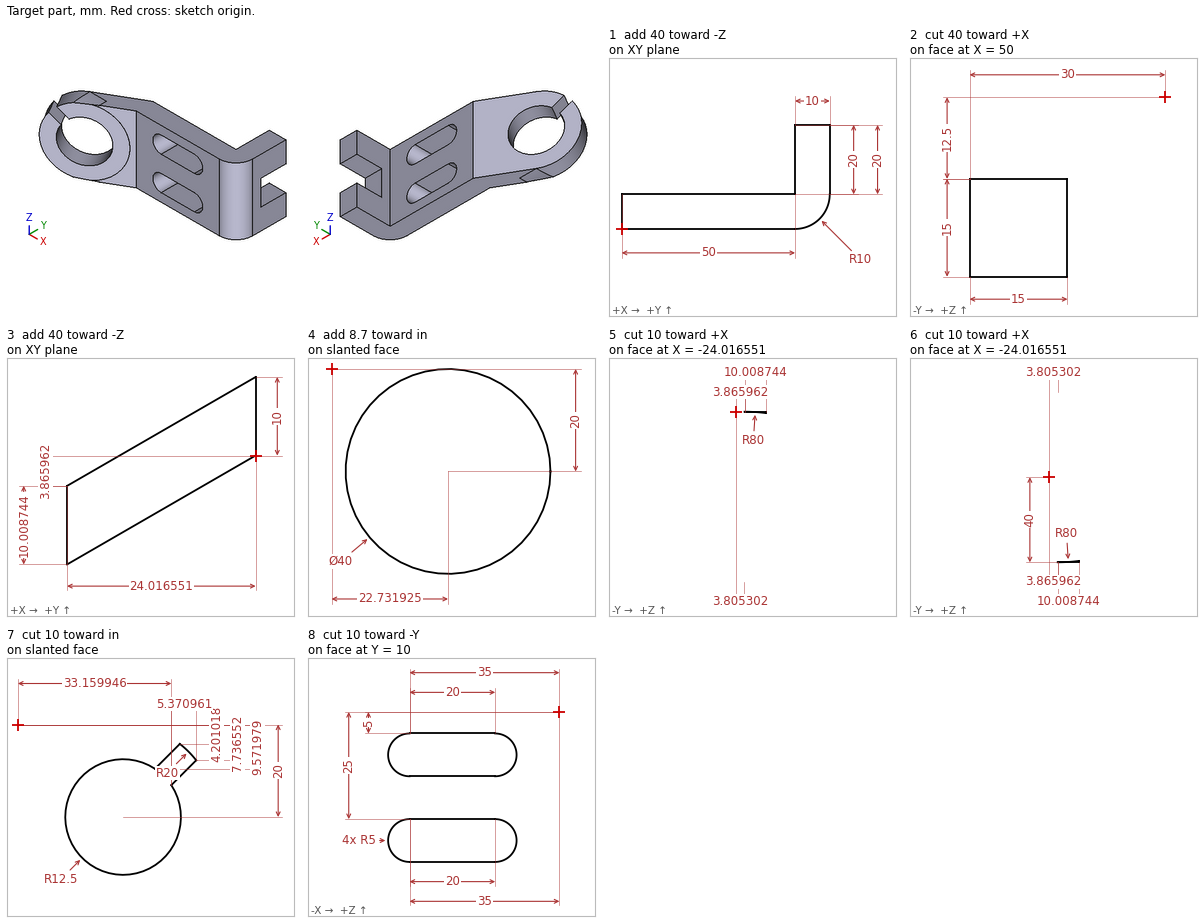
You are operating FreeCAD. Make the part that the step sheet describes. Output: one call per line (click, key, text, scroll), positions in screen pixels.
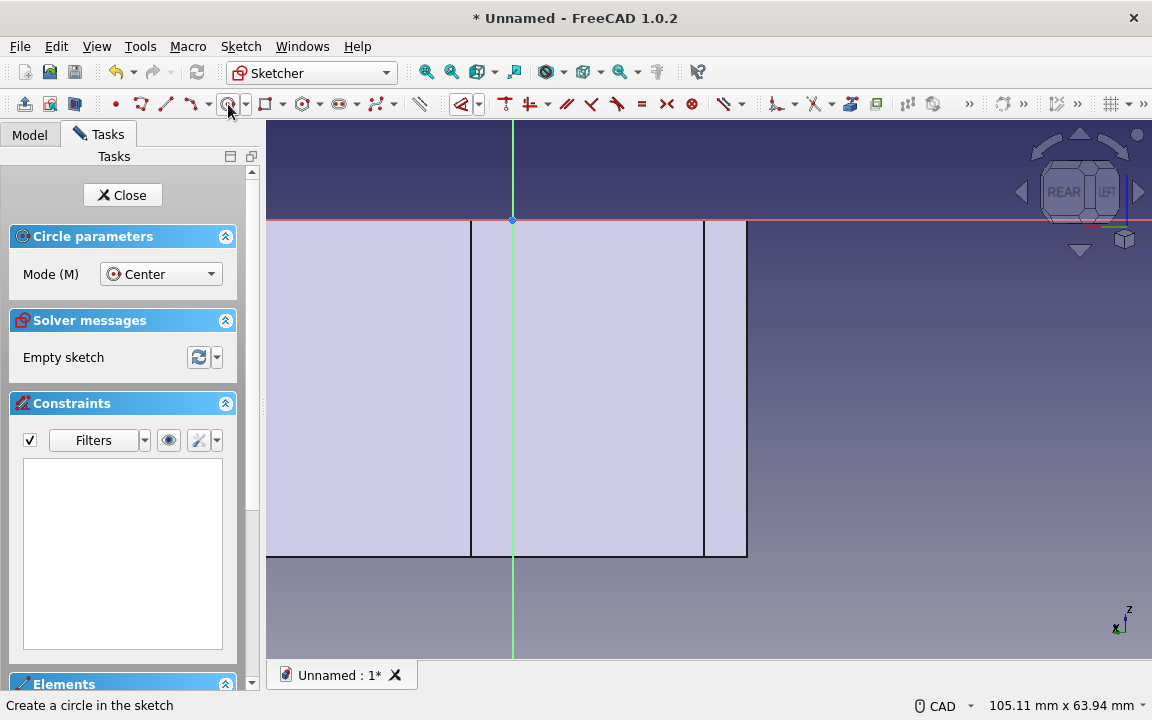
click(704, 389)
click(824, 269)
key(Escape)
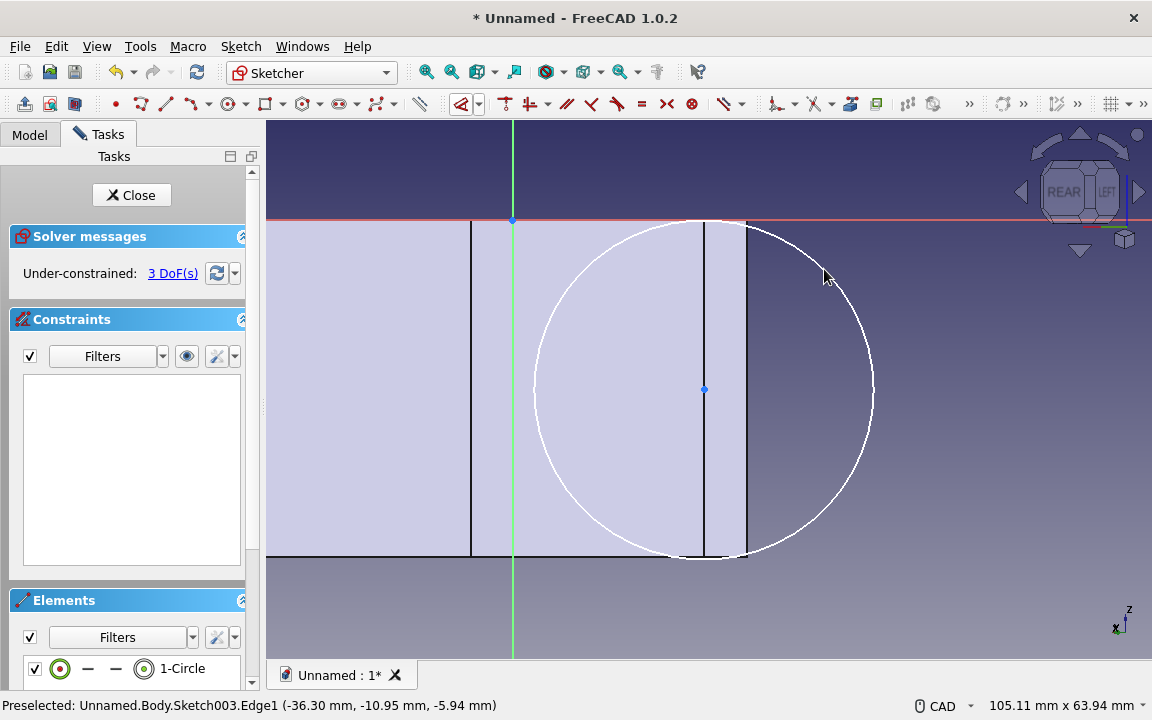
click(824, 270)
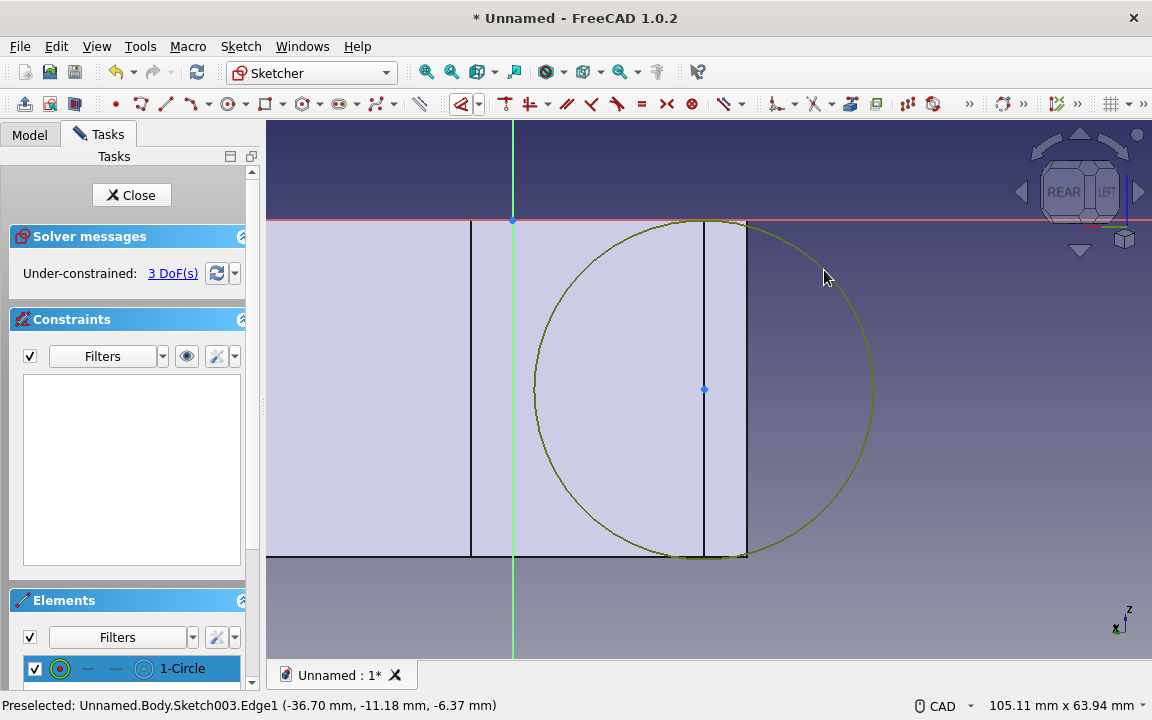
key(k)
key(o)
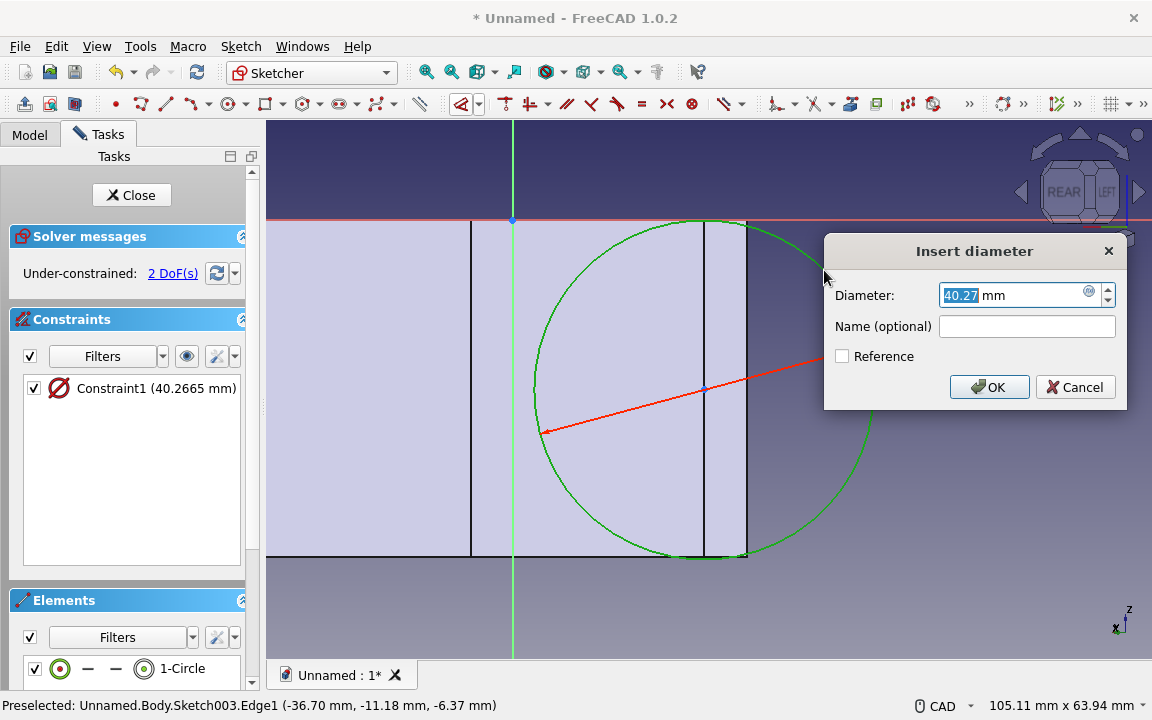
text(40)
key(Return)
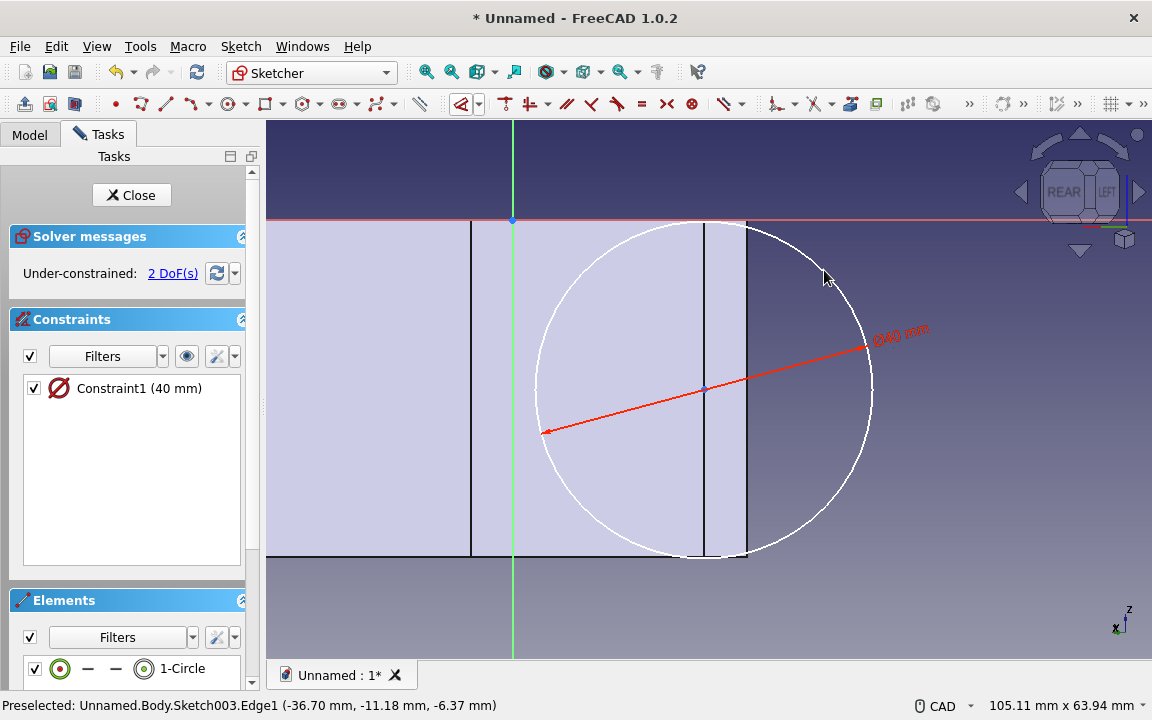
click(704, 390)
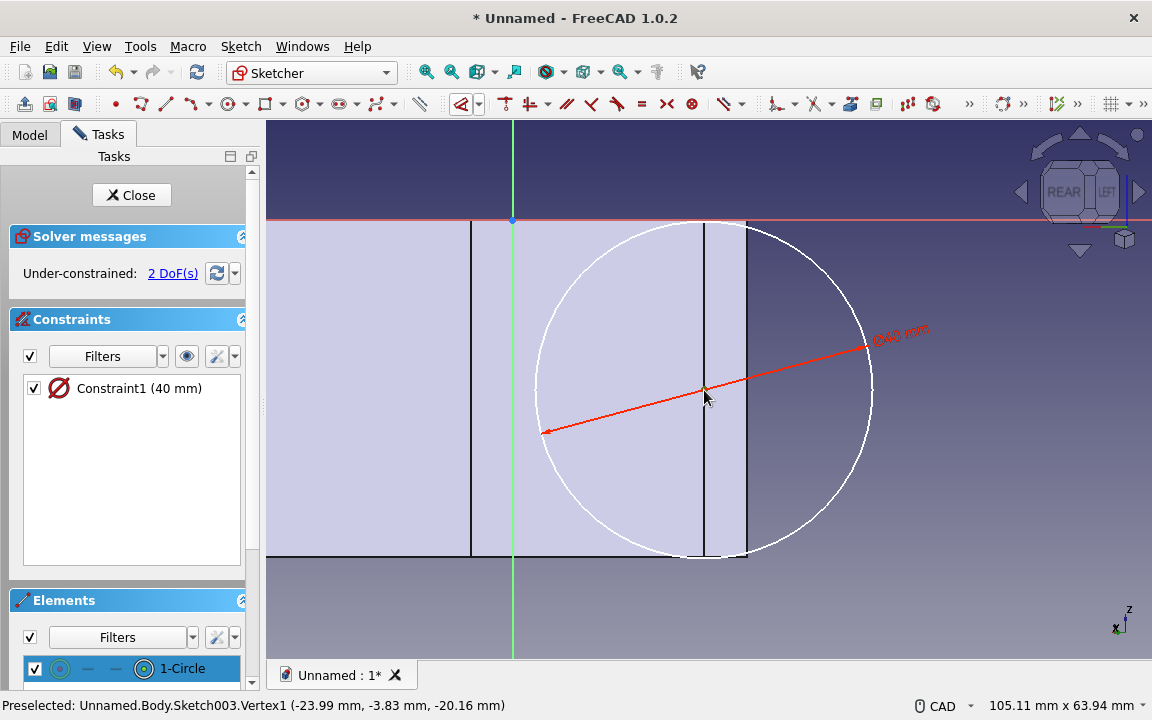
key(i)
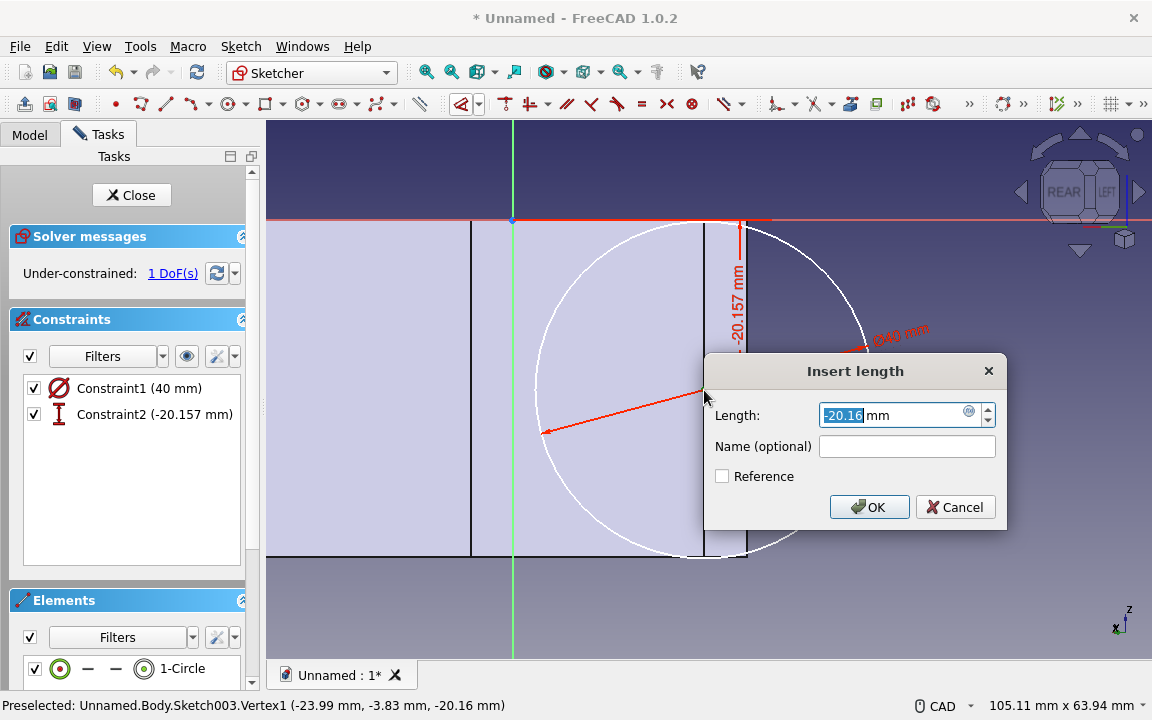
text(-20)
key(Return)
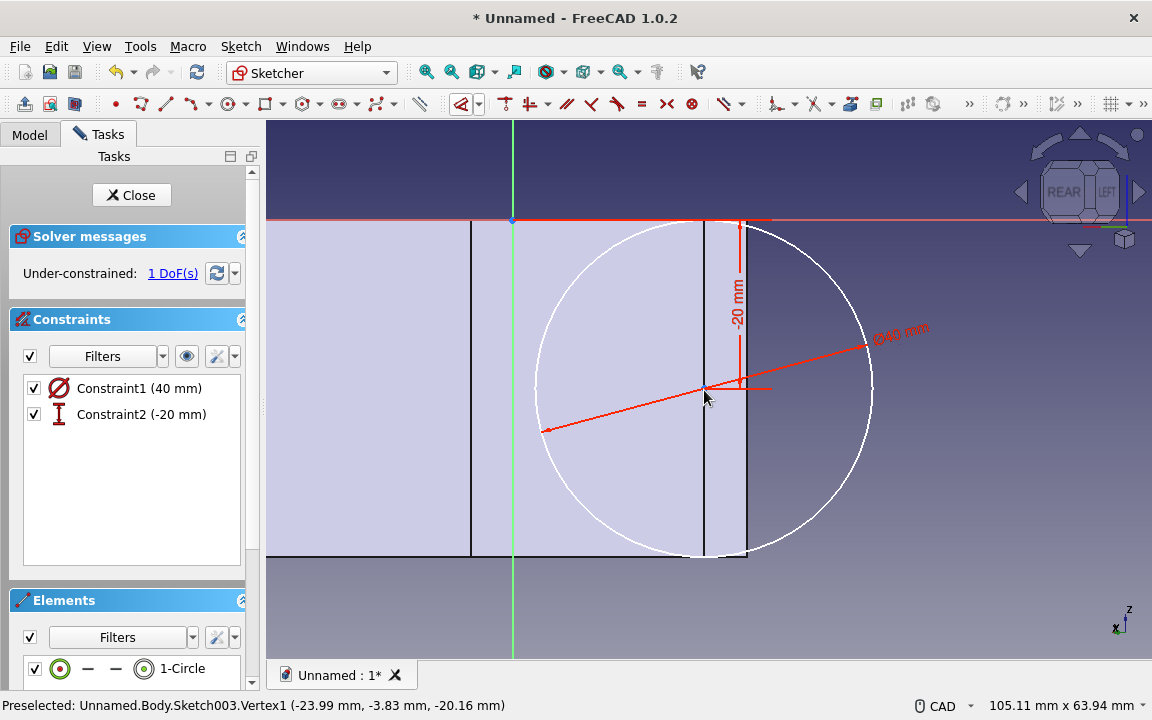
click(704, 389)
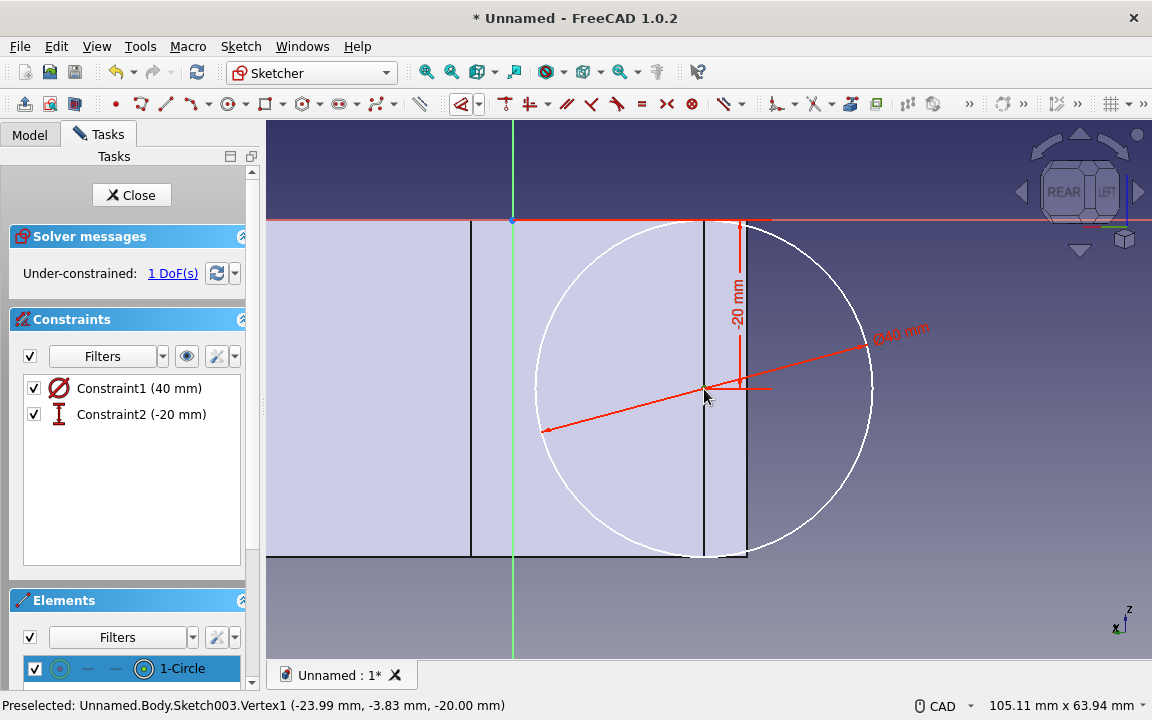
key(l)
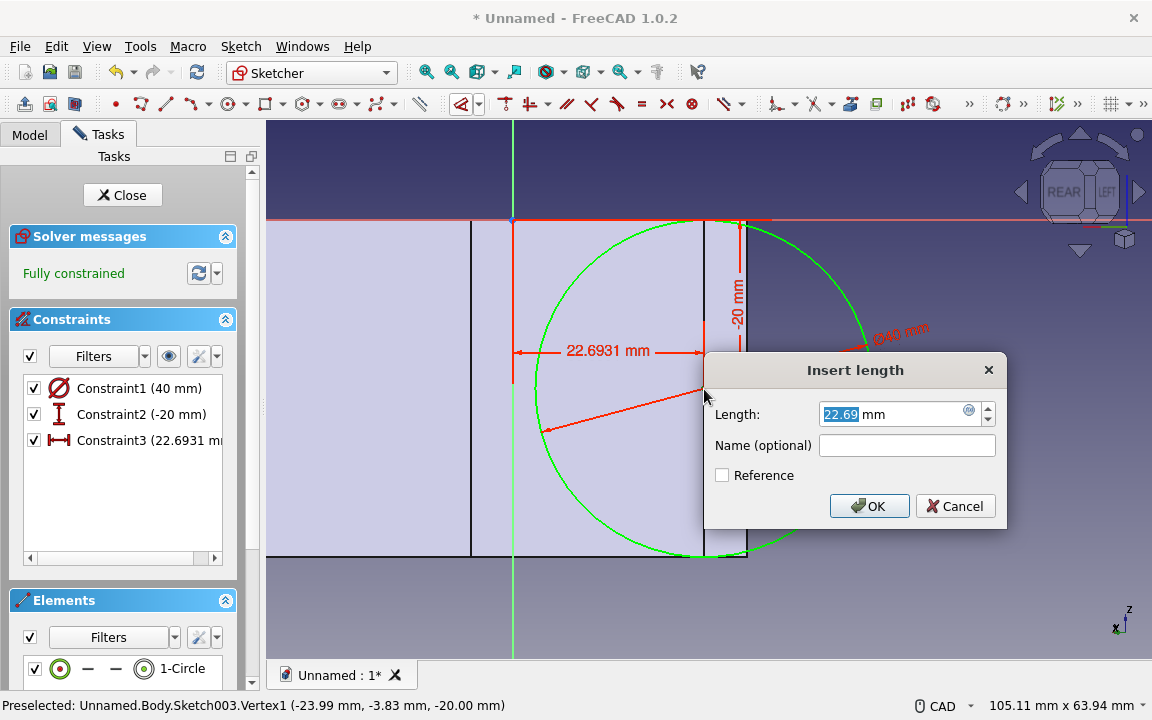
text(22.731925)
key(Return)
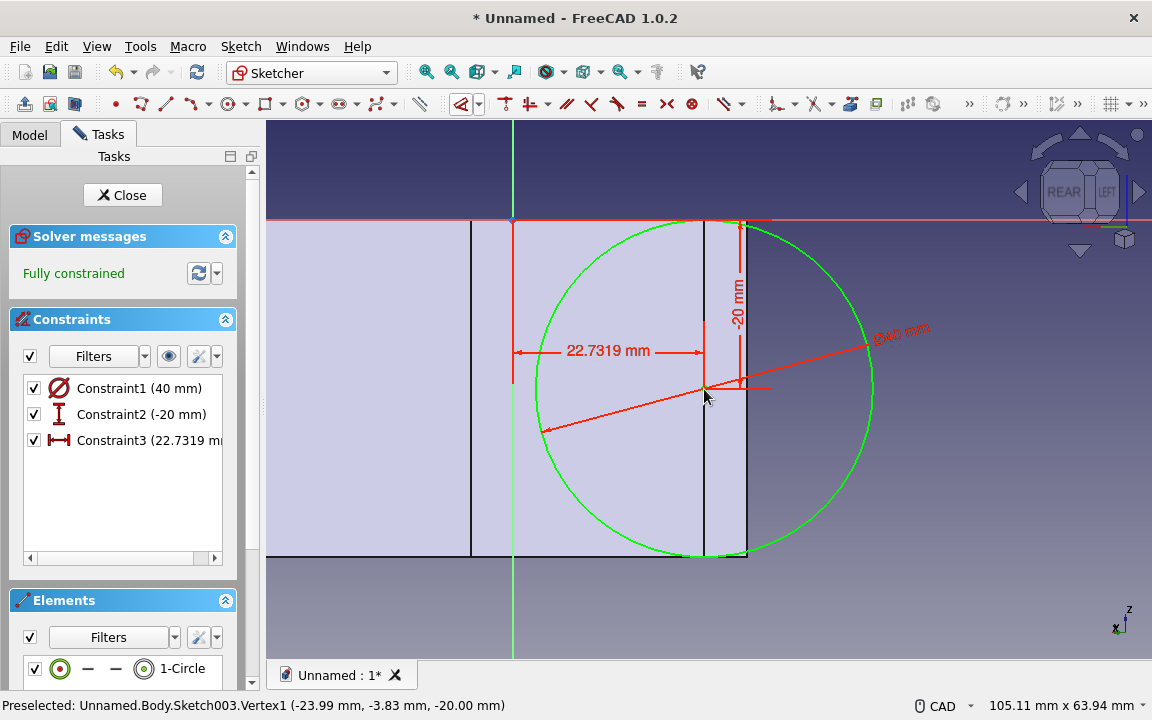
click(123, 195)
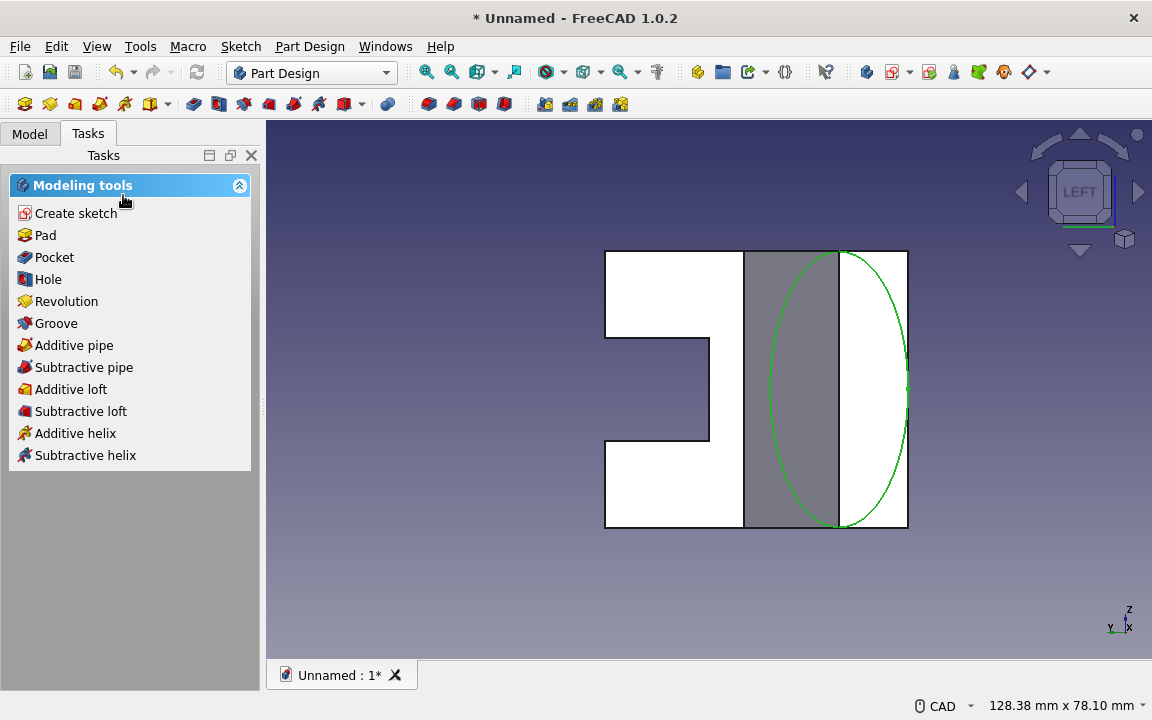
click(25, 104)